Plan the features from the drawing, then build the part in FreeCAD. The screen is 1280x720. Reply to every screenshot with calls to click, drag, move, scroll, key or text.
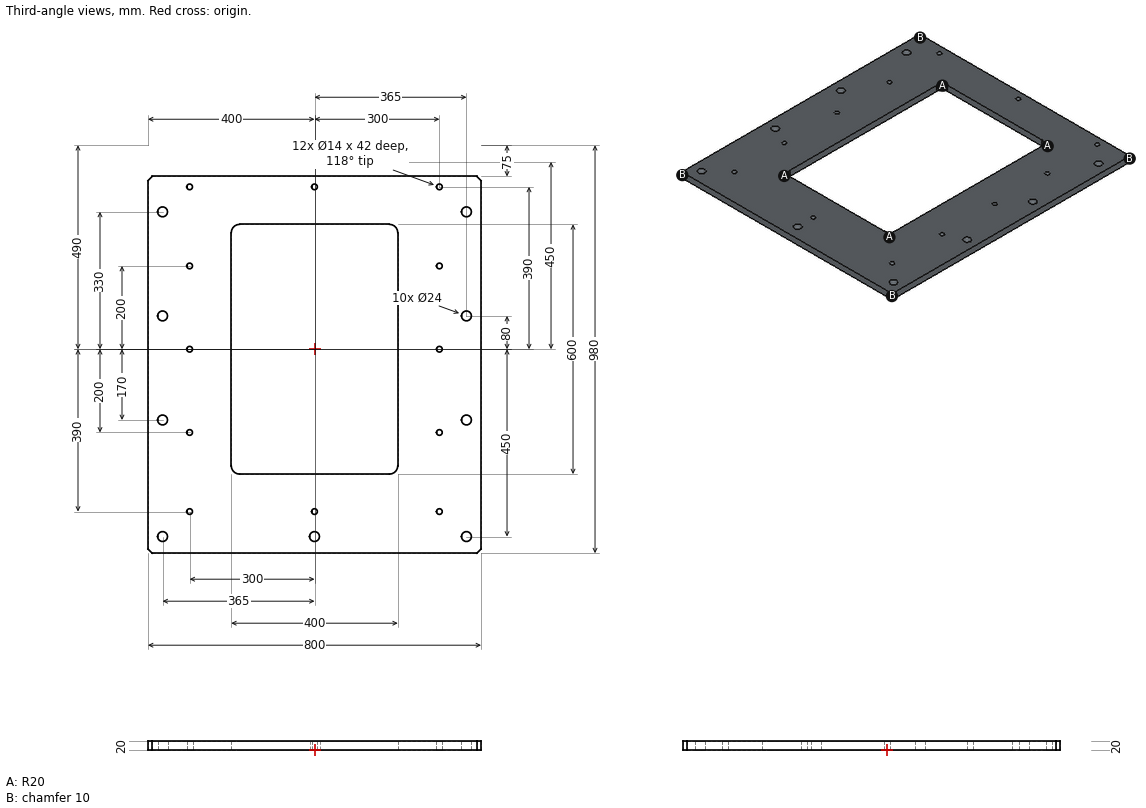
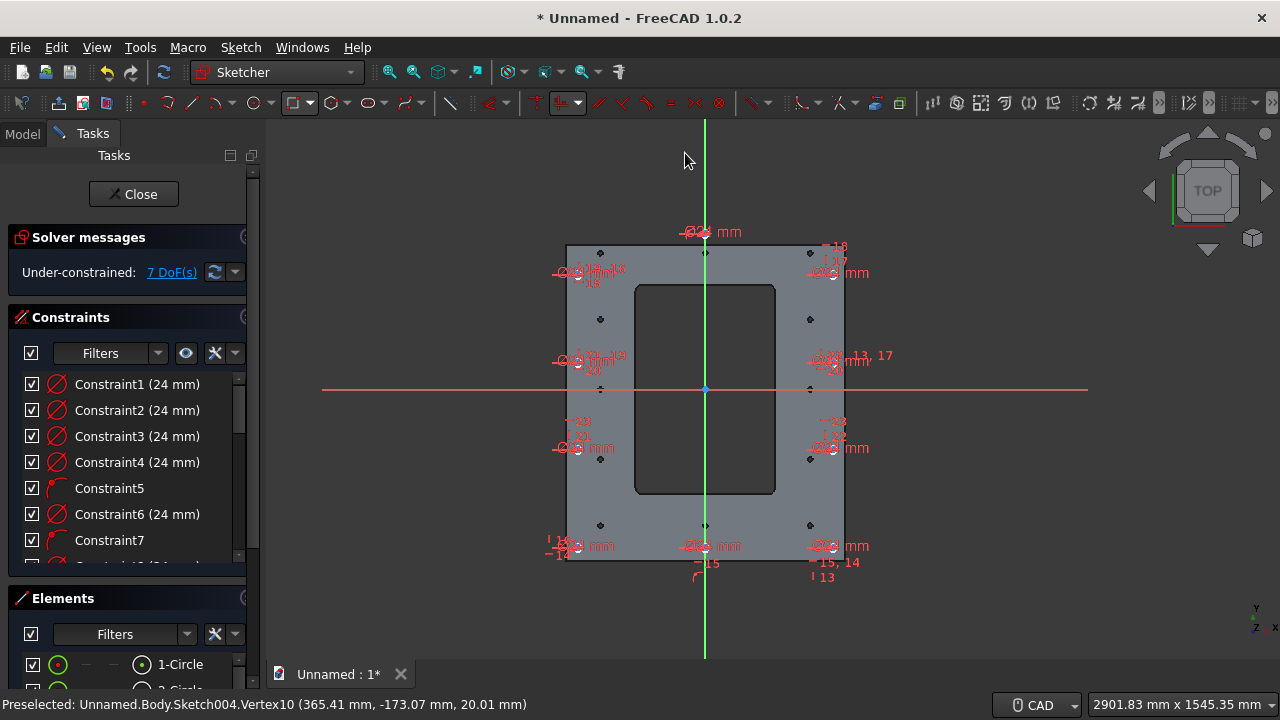
click(490, 104)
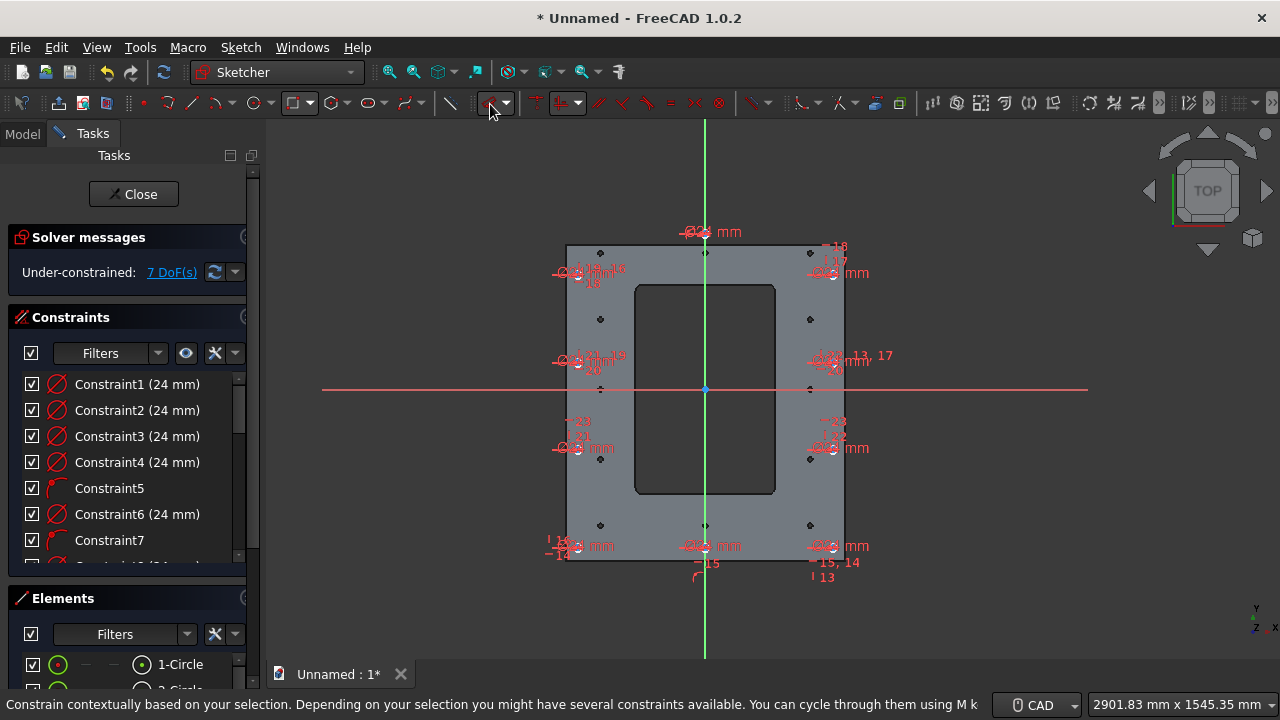
scroll(833, 363, up, 2)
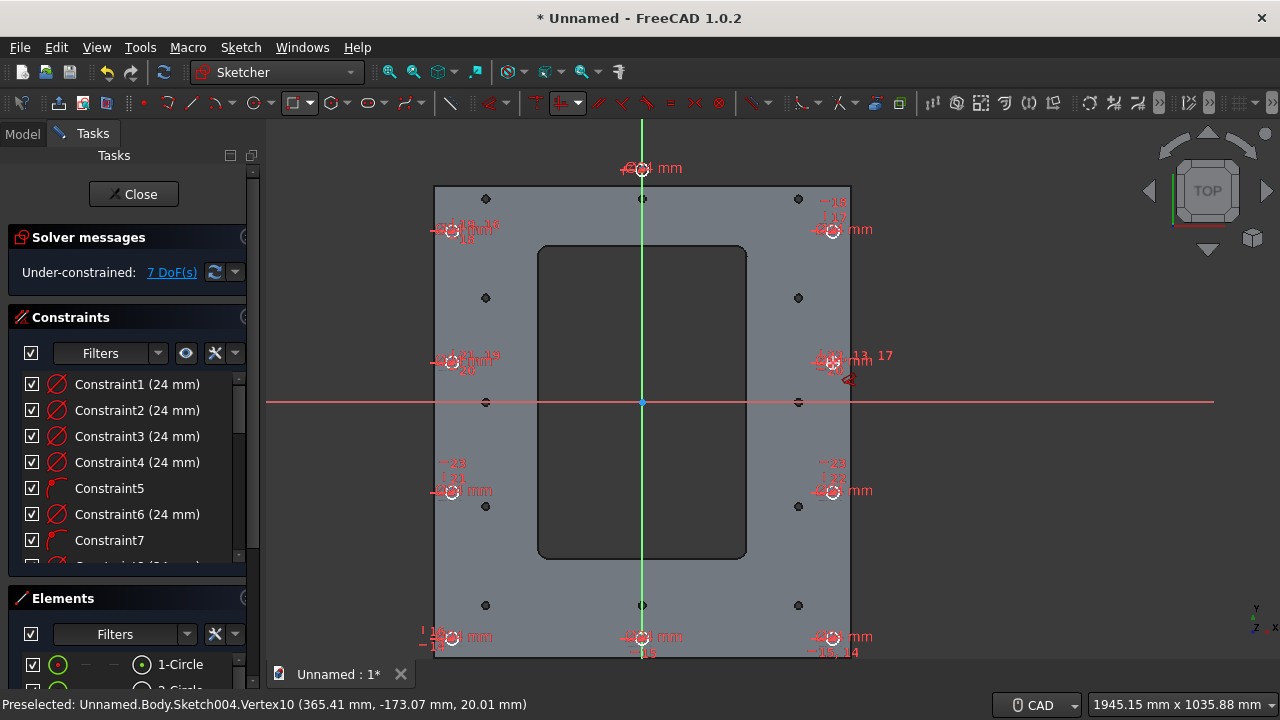
click(833, 363)
click(867, 383)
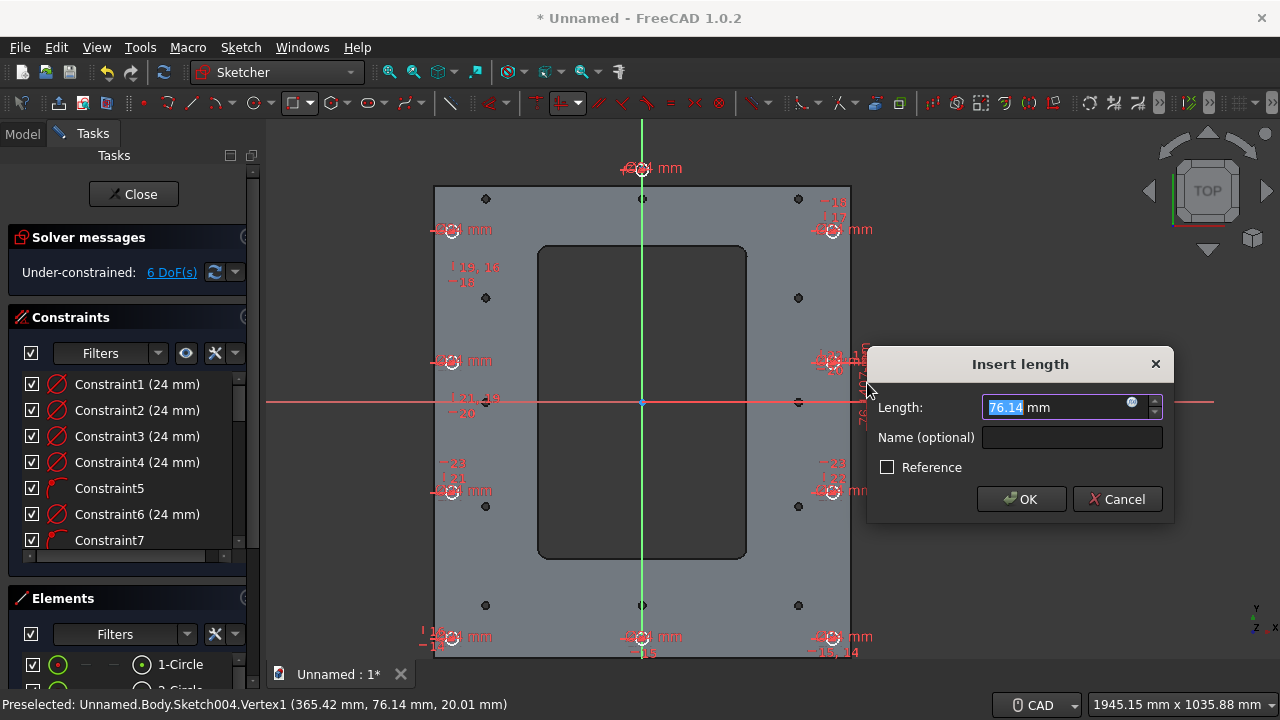
text(80)
key(Return)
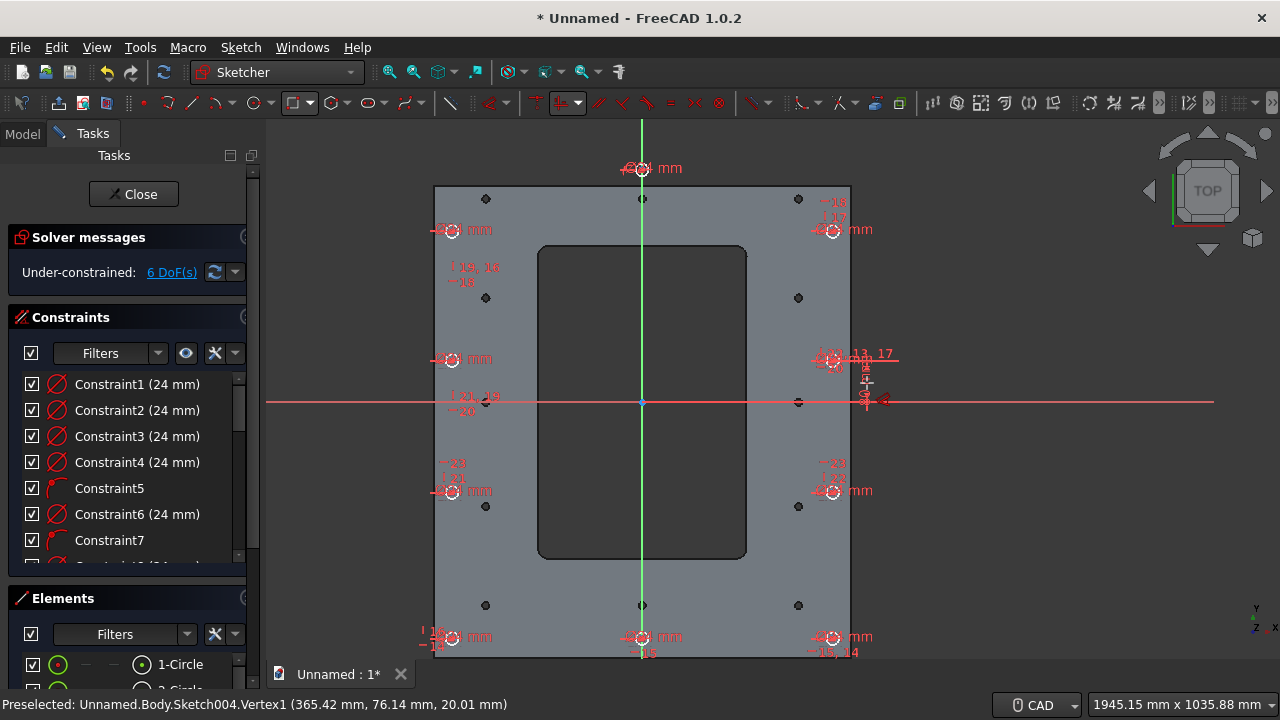
click(833, 361)
click(737, 327)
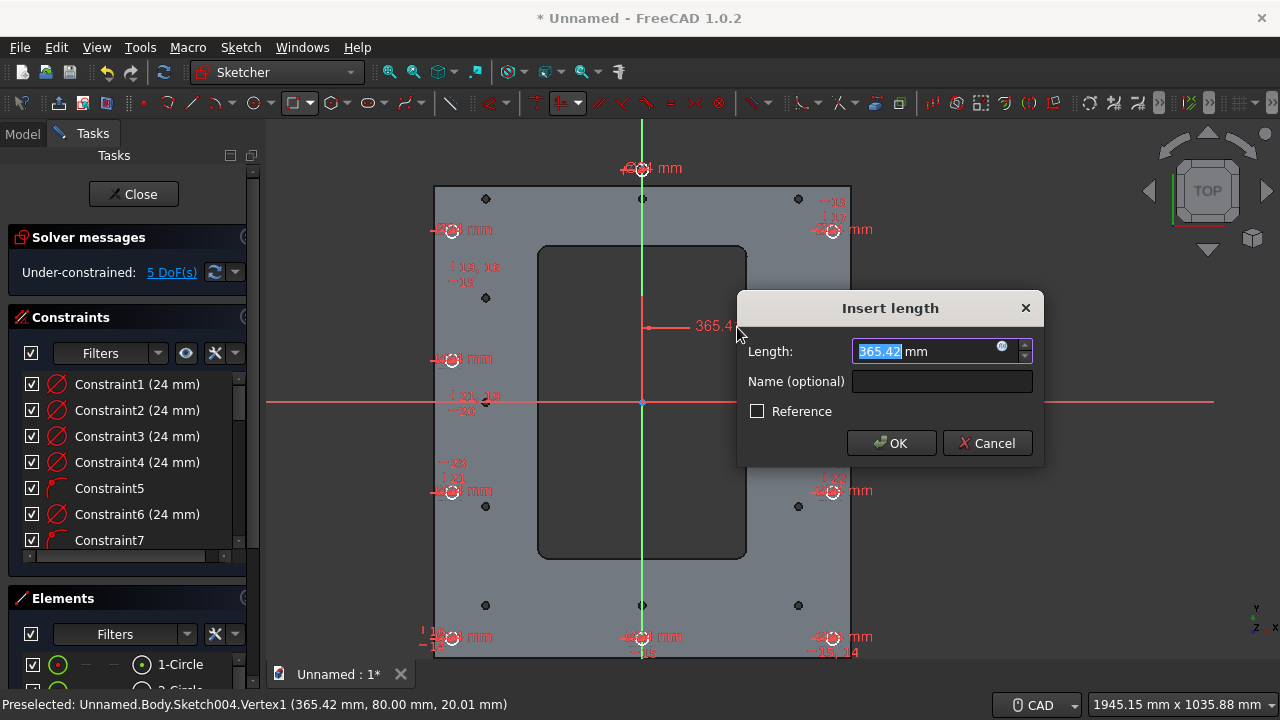
text(365)
key(Return)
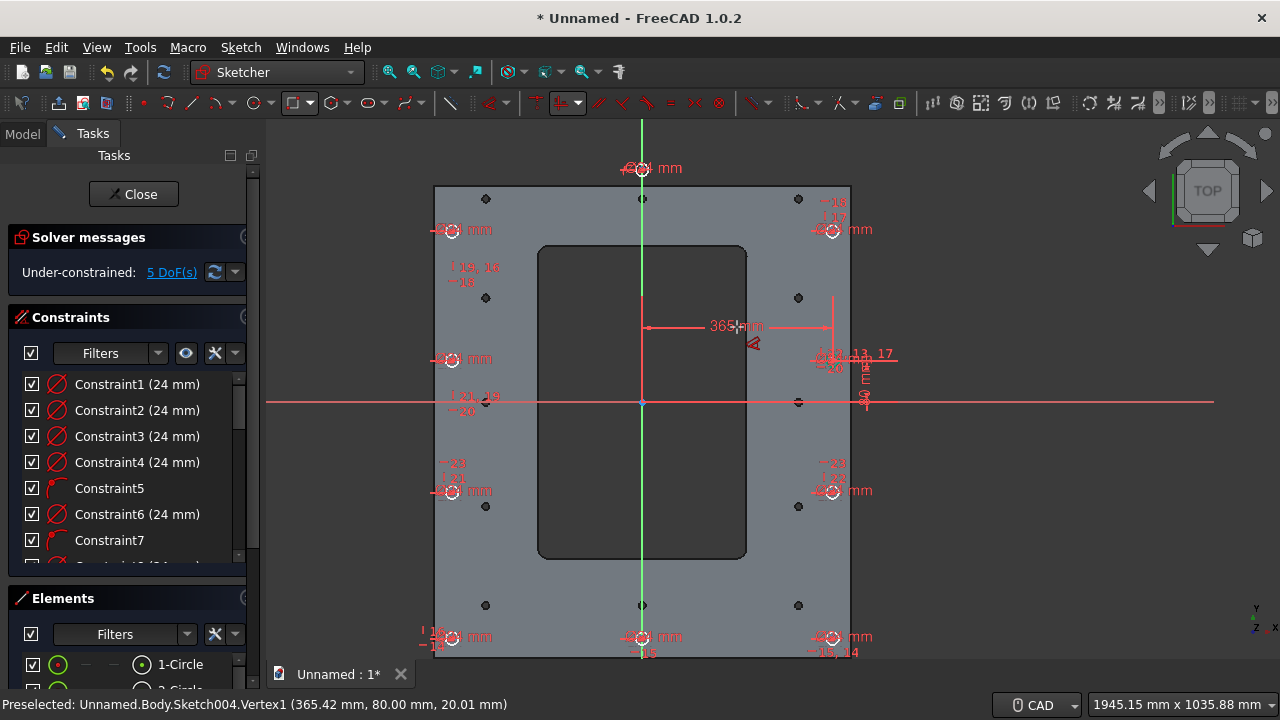
scroll(831, 362, down, 2)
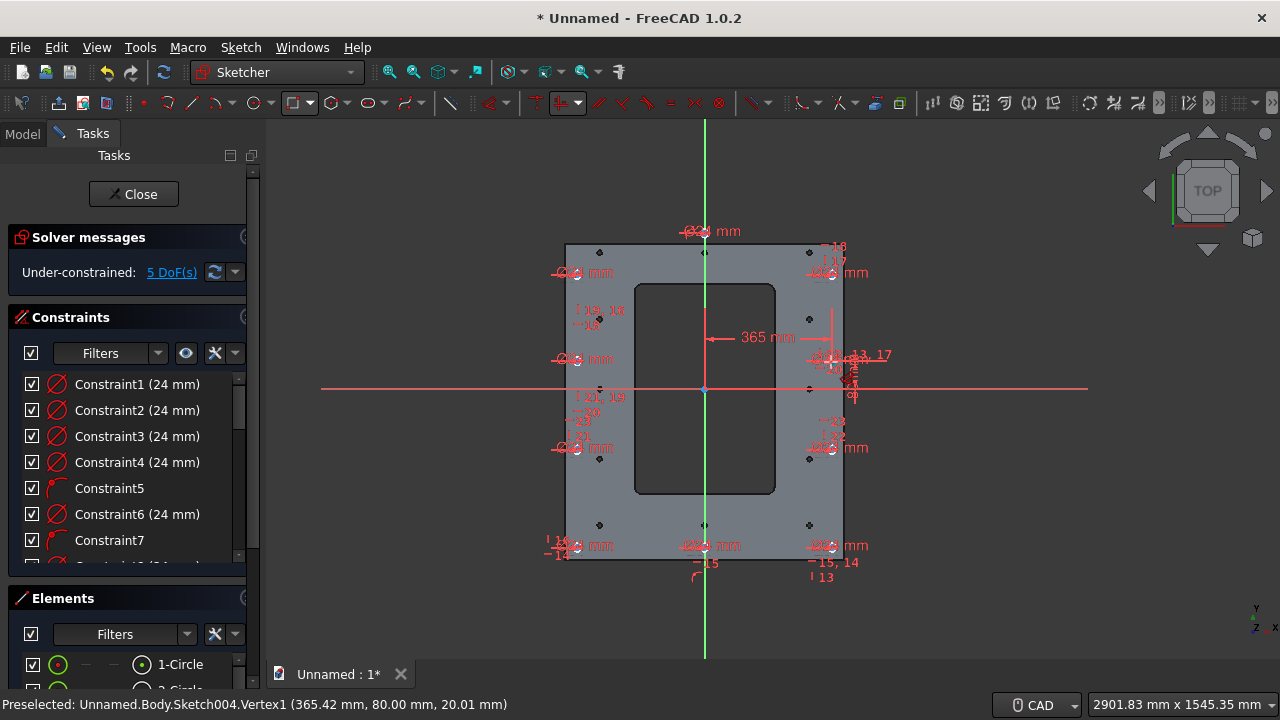
click(832, 548)
click(866, 468)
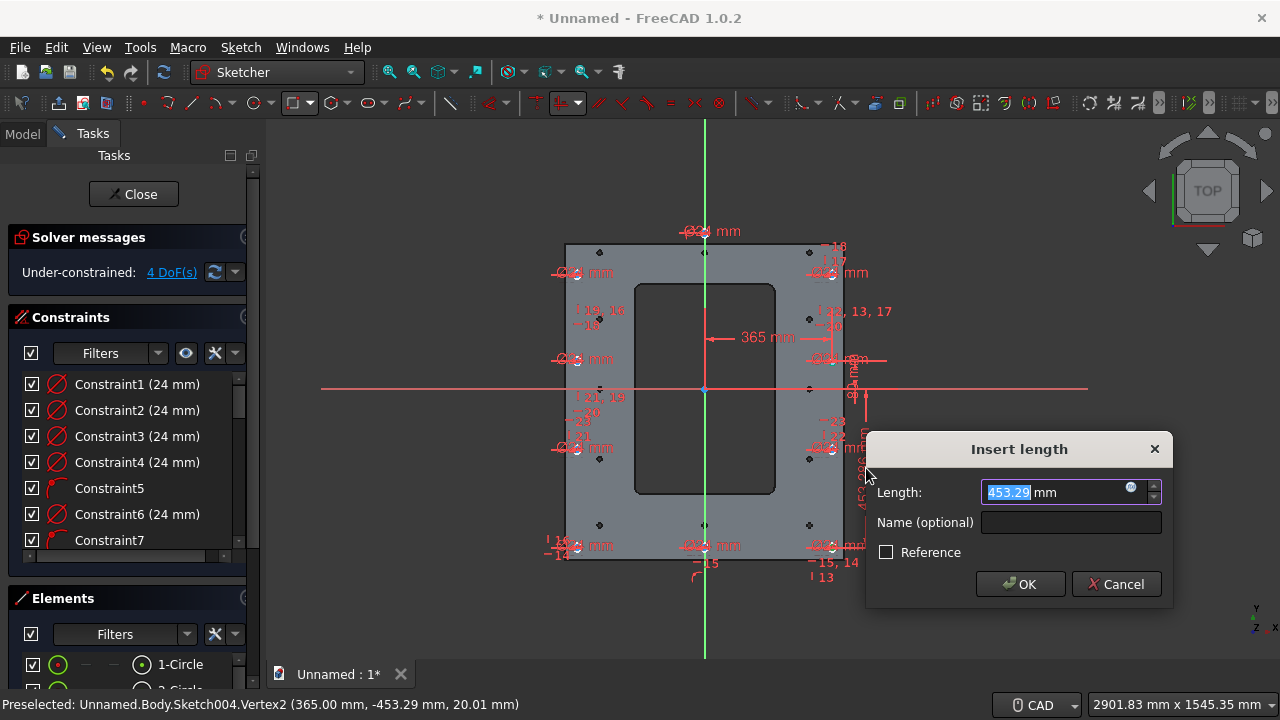
text(450)
key(Return)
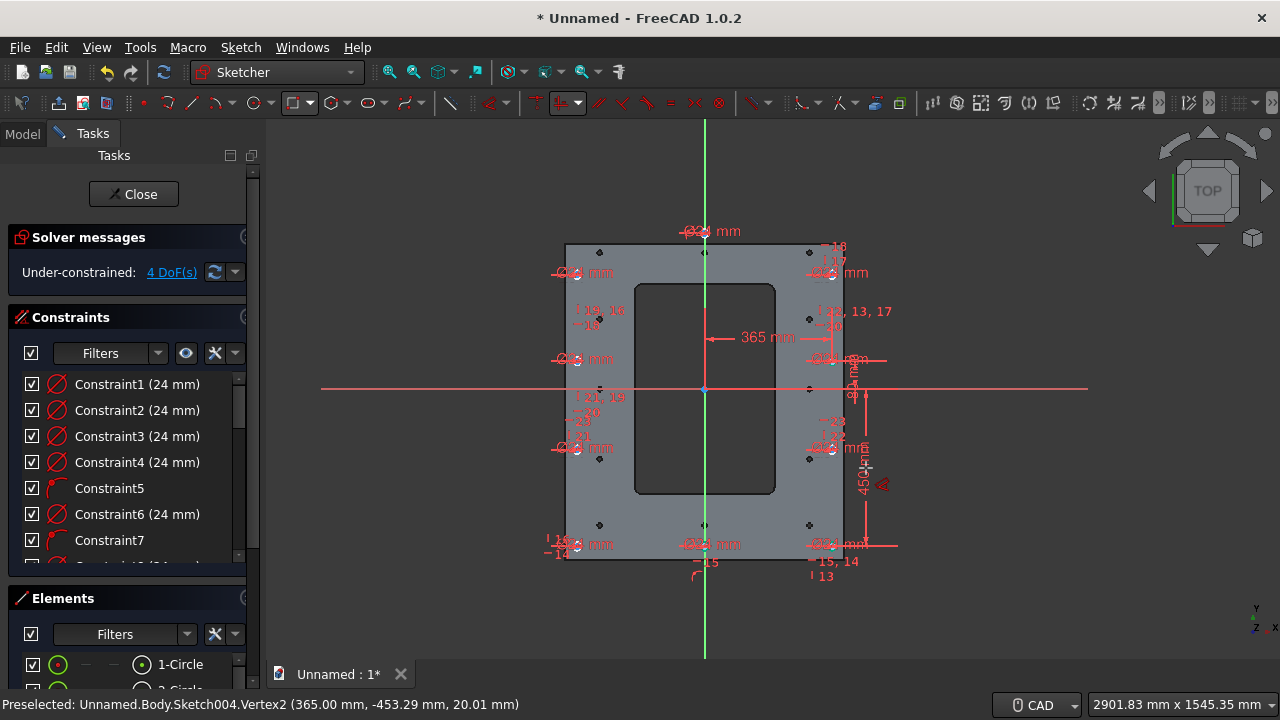
click(577, 546)
click(641, 580)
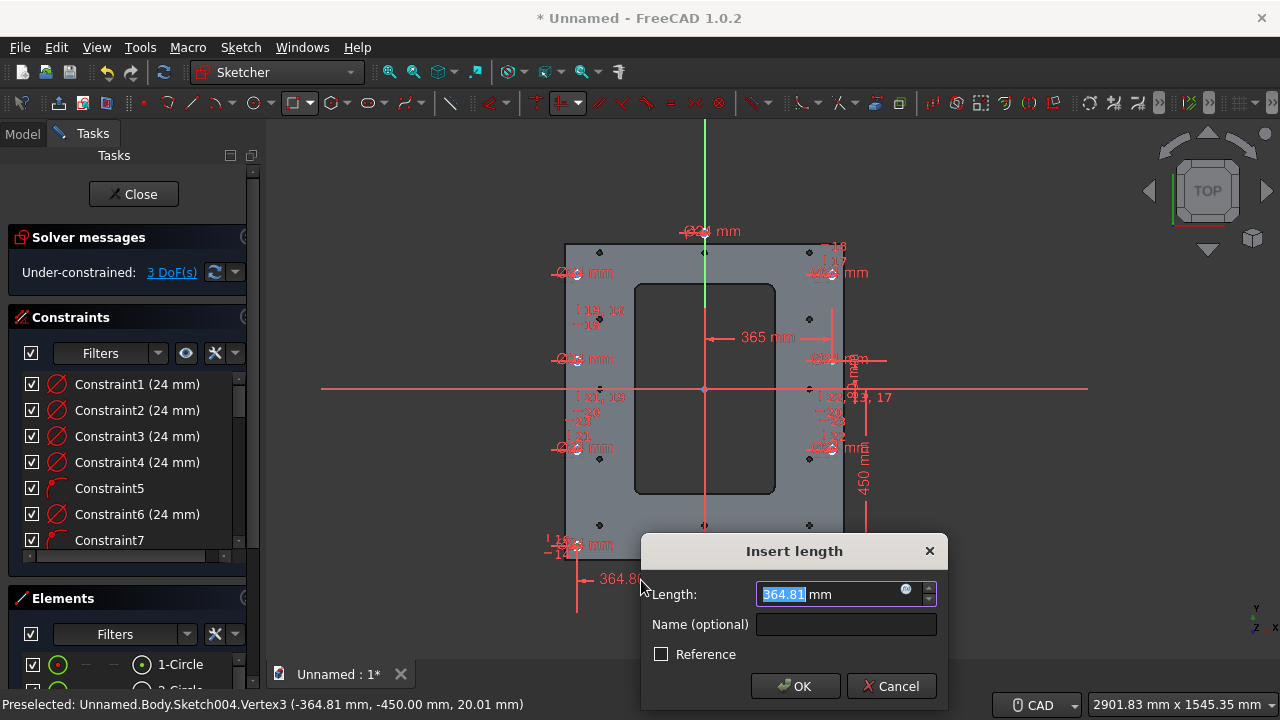
text(365)
key(Return)